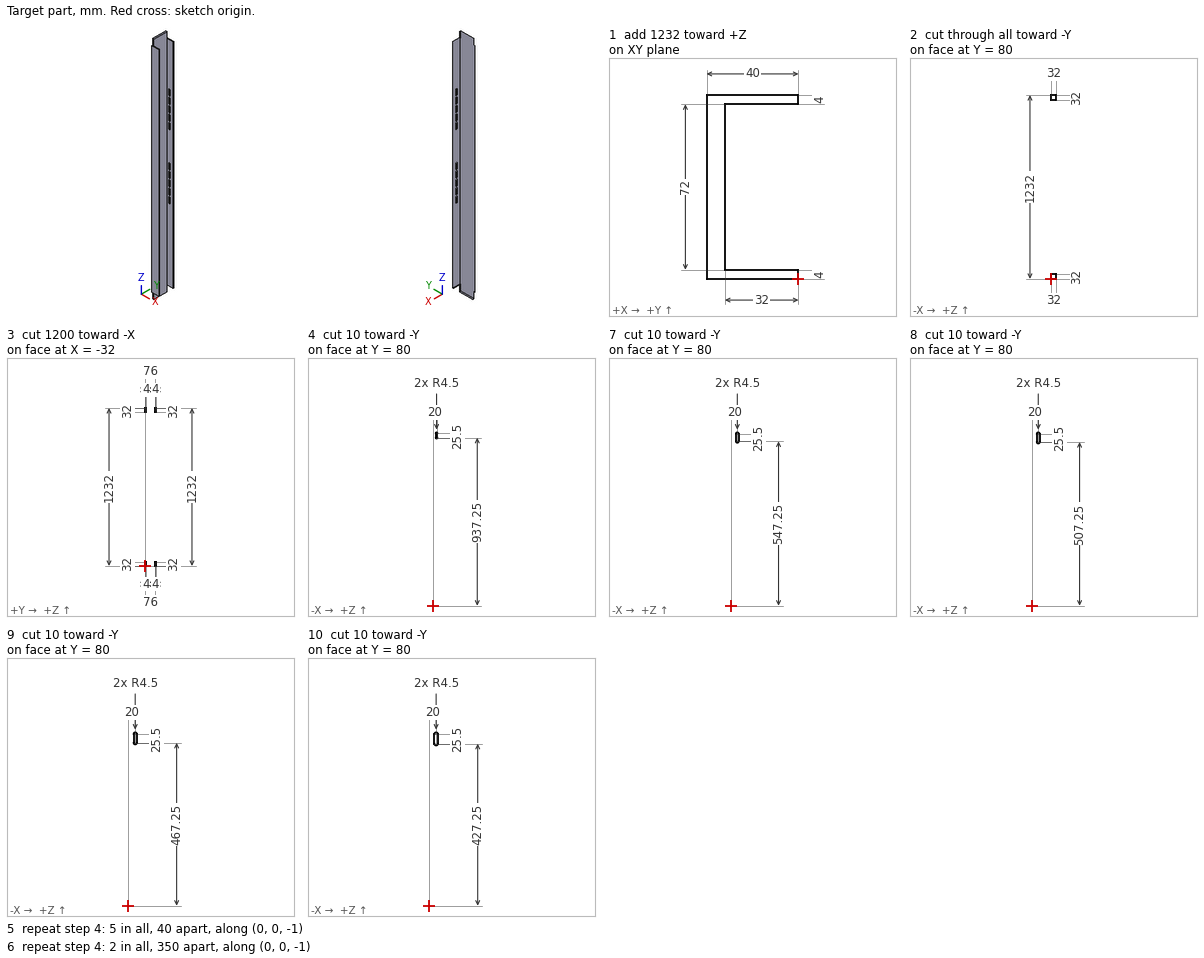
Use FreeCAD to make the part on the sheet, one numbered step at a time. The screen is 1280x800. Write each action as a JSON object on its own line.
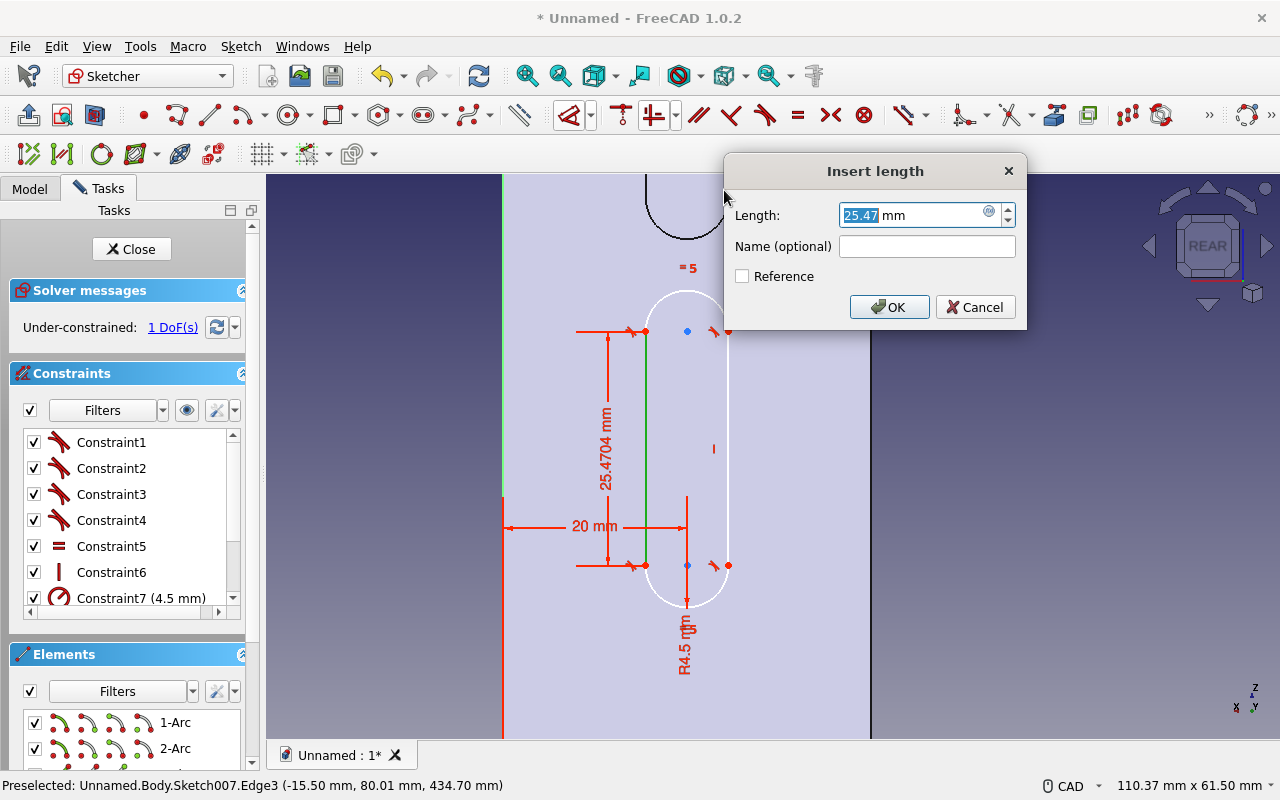
{"action": "type", "text": "25.5"}
{"action": "key", "text": "Return"}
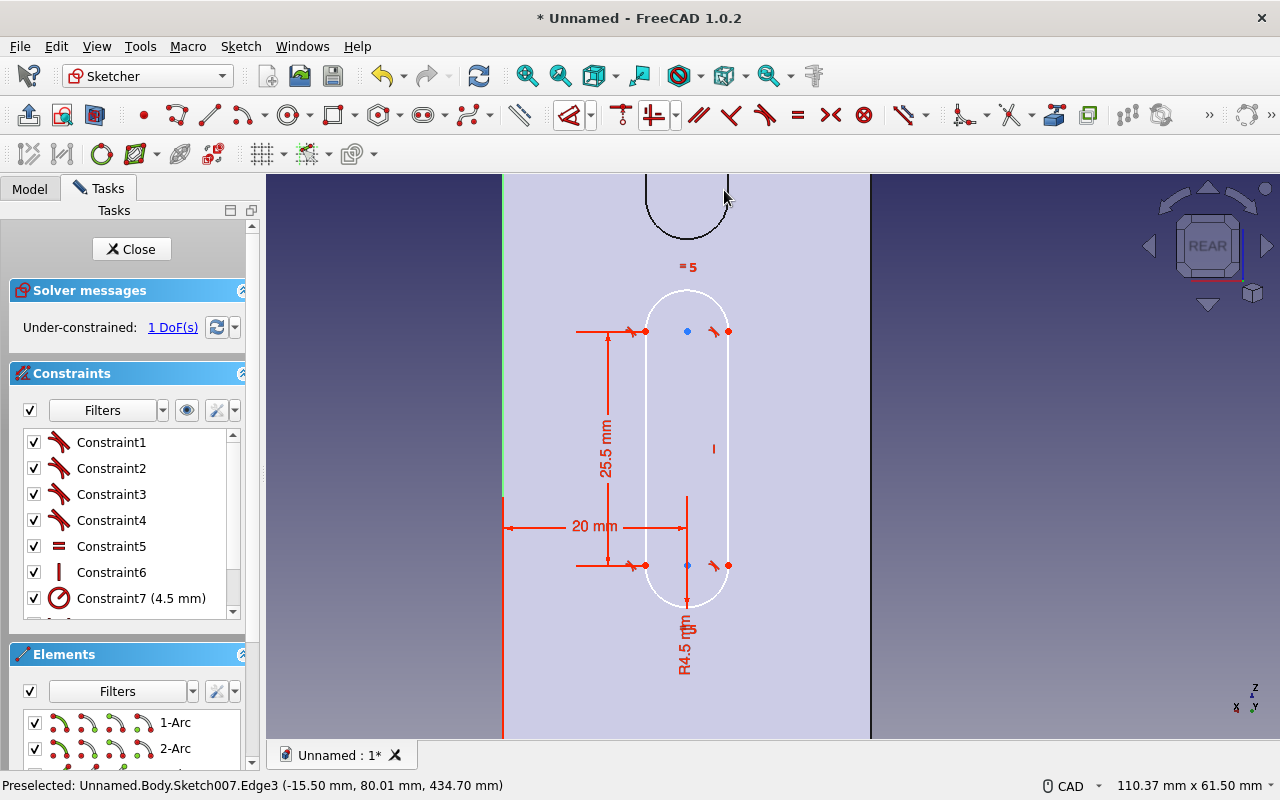
{"action": "left_click", "coordinate": [646, 566]}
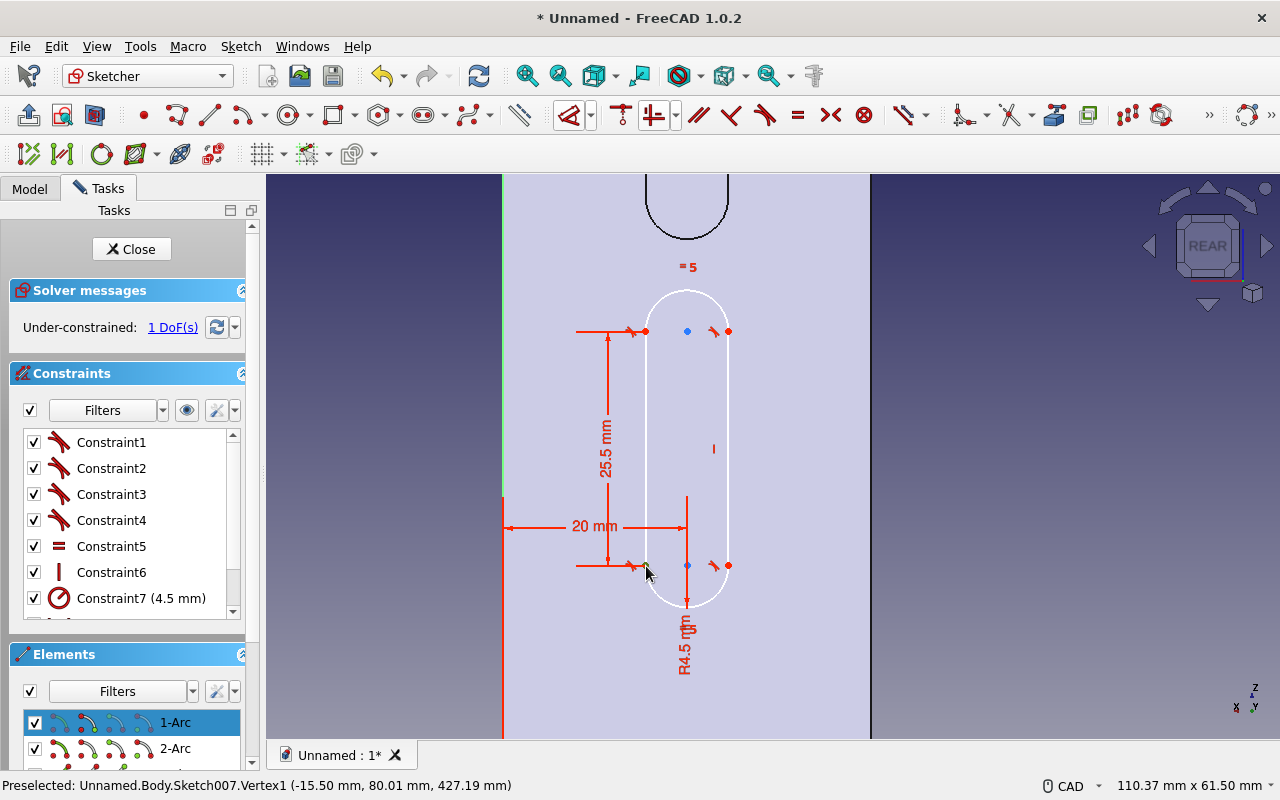
{"action": "left_click", "coordinate": [590, 116]}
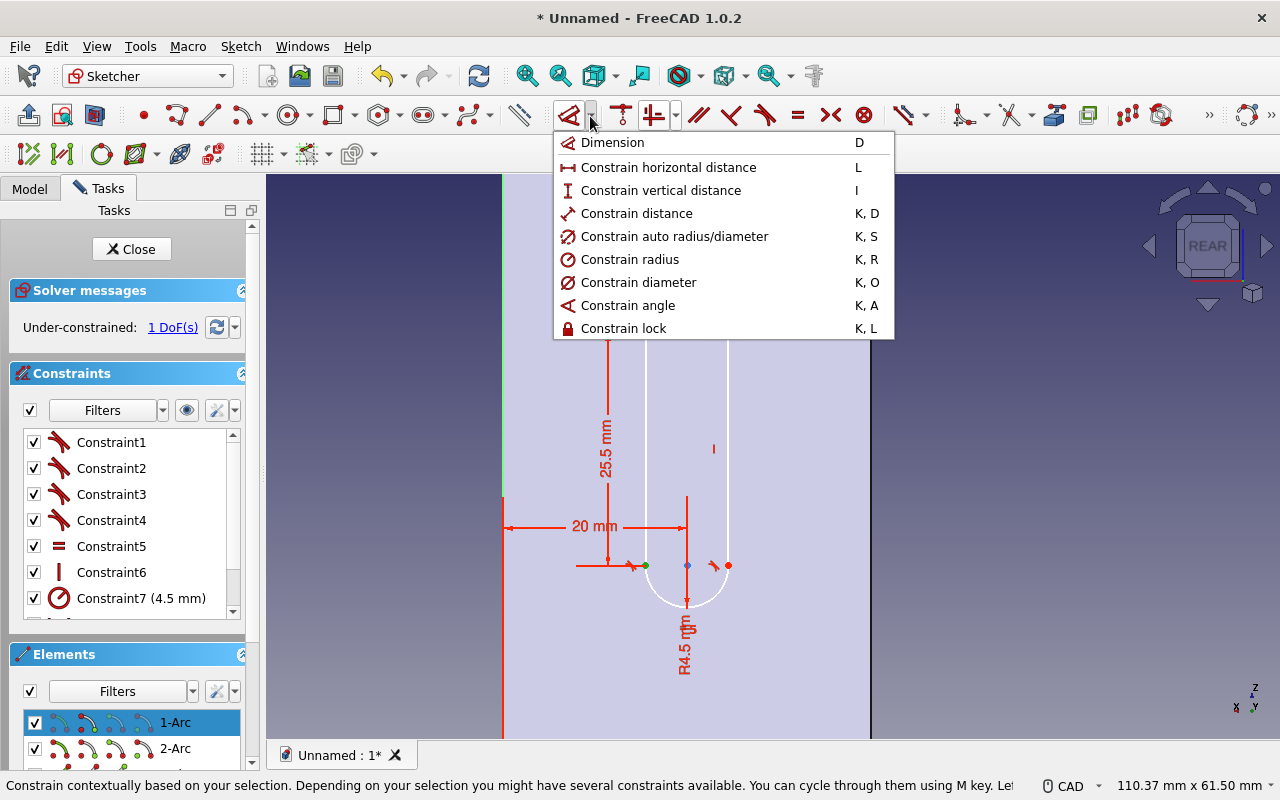
{"action": "left_click", "coordinate": [724, 190]}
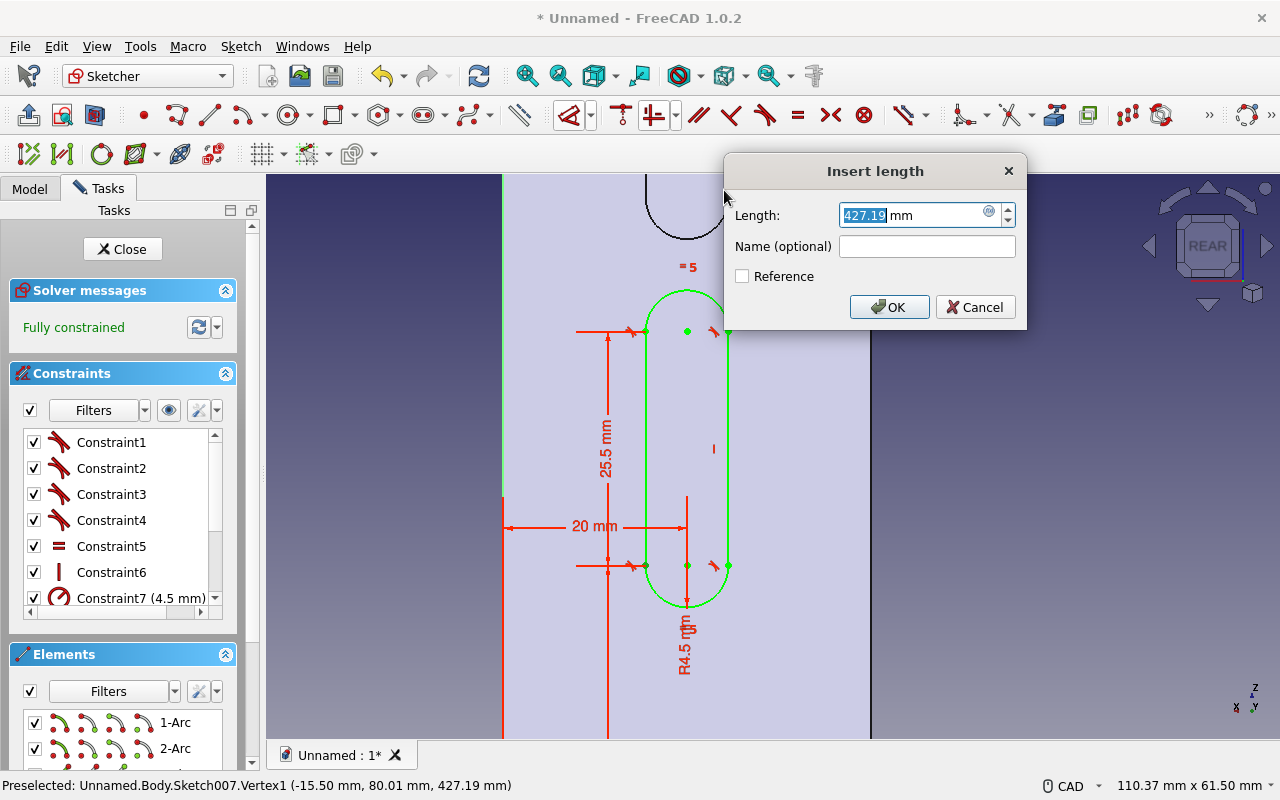
{"action": "type", "text": "427.25"}
{"action": "key", "text": "Return"}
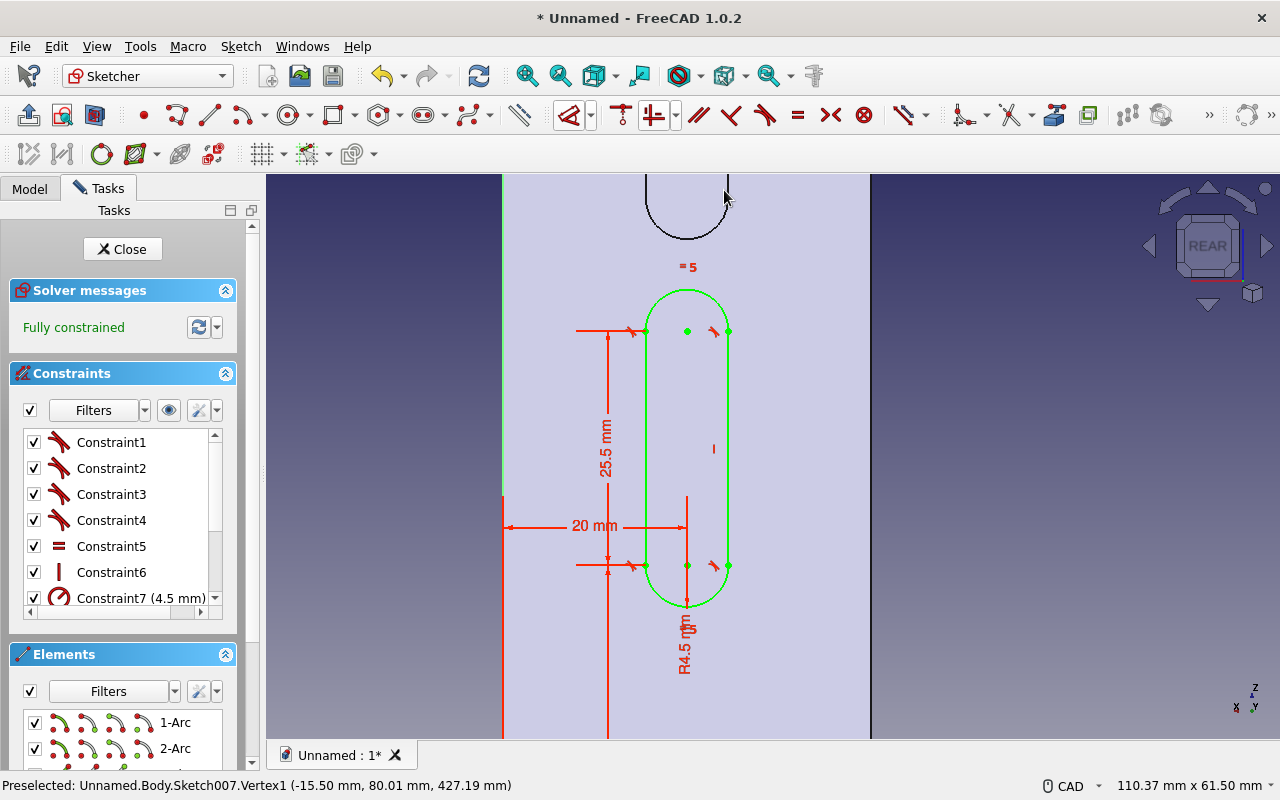
{"action": "left_click", "coordinate": [123, 249]}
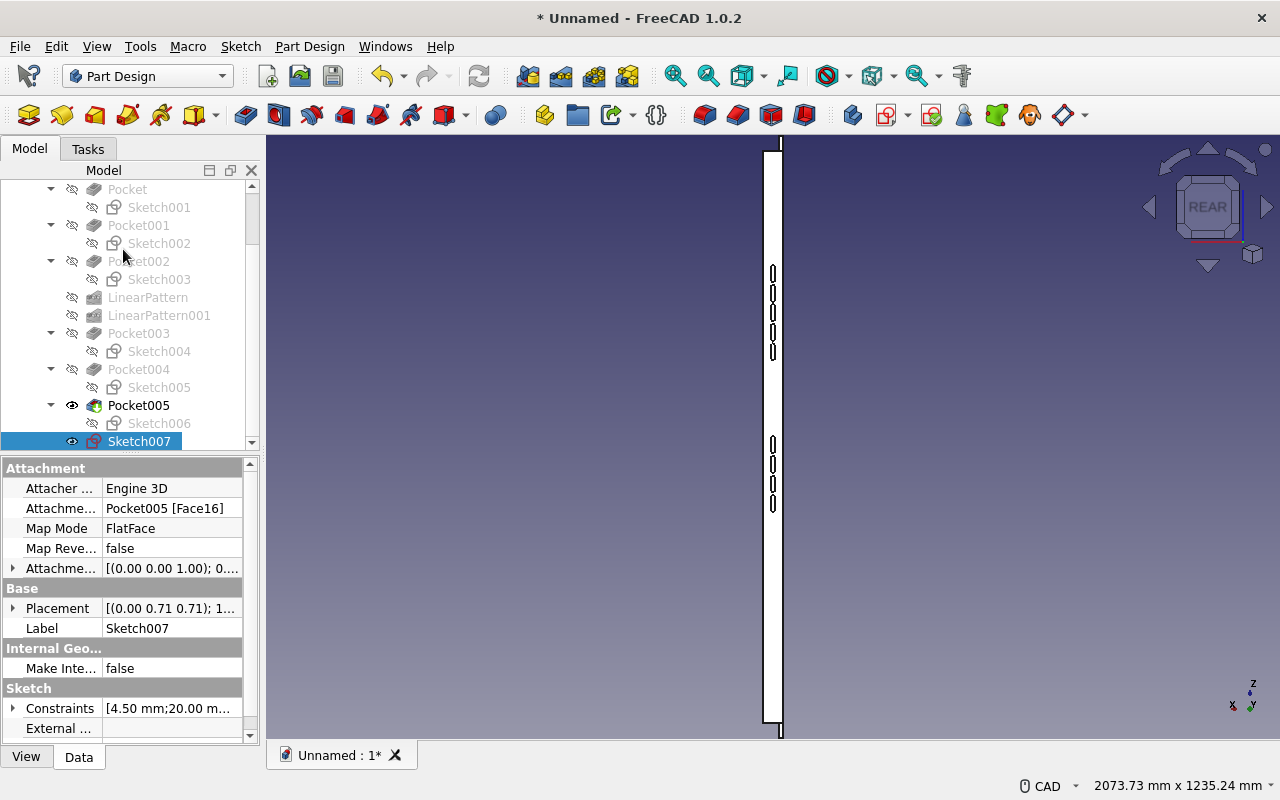
{"action": "left_click", "coordinate": [246, 116]}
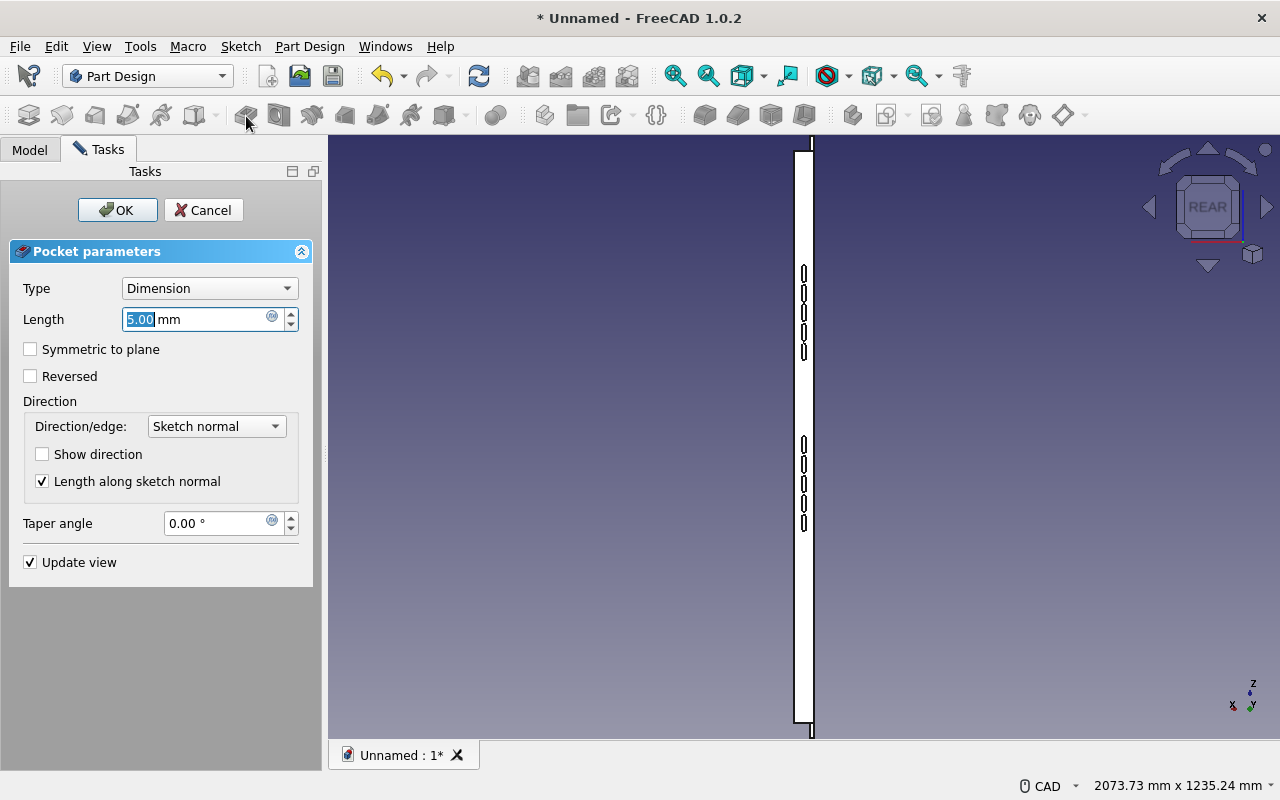
{"action": "type", "text": "10"}
{"action": "key", "text": "Tab"}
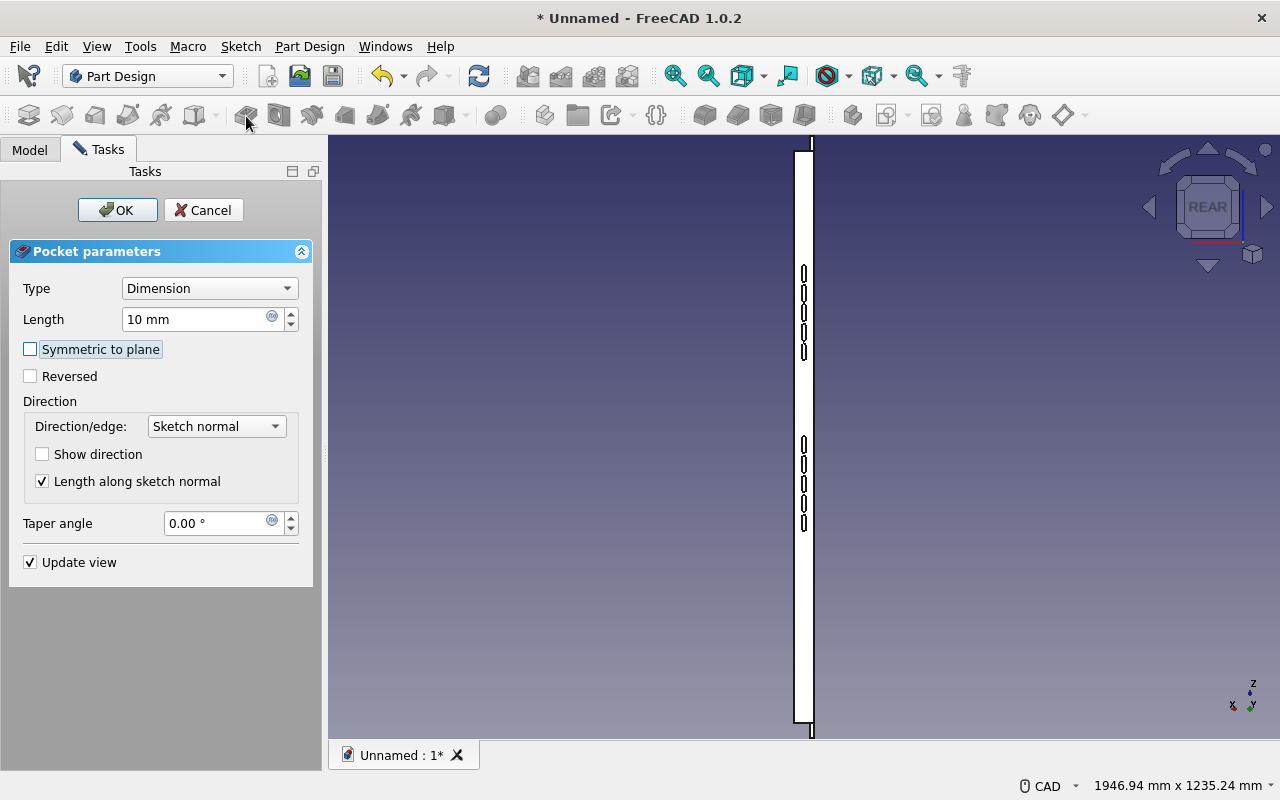
{"action": "left_click", "coordinate": [118, 210]}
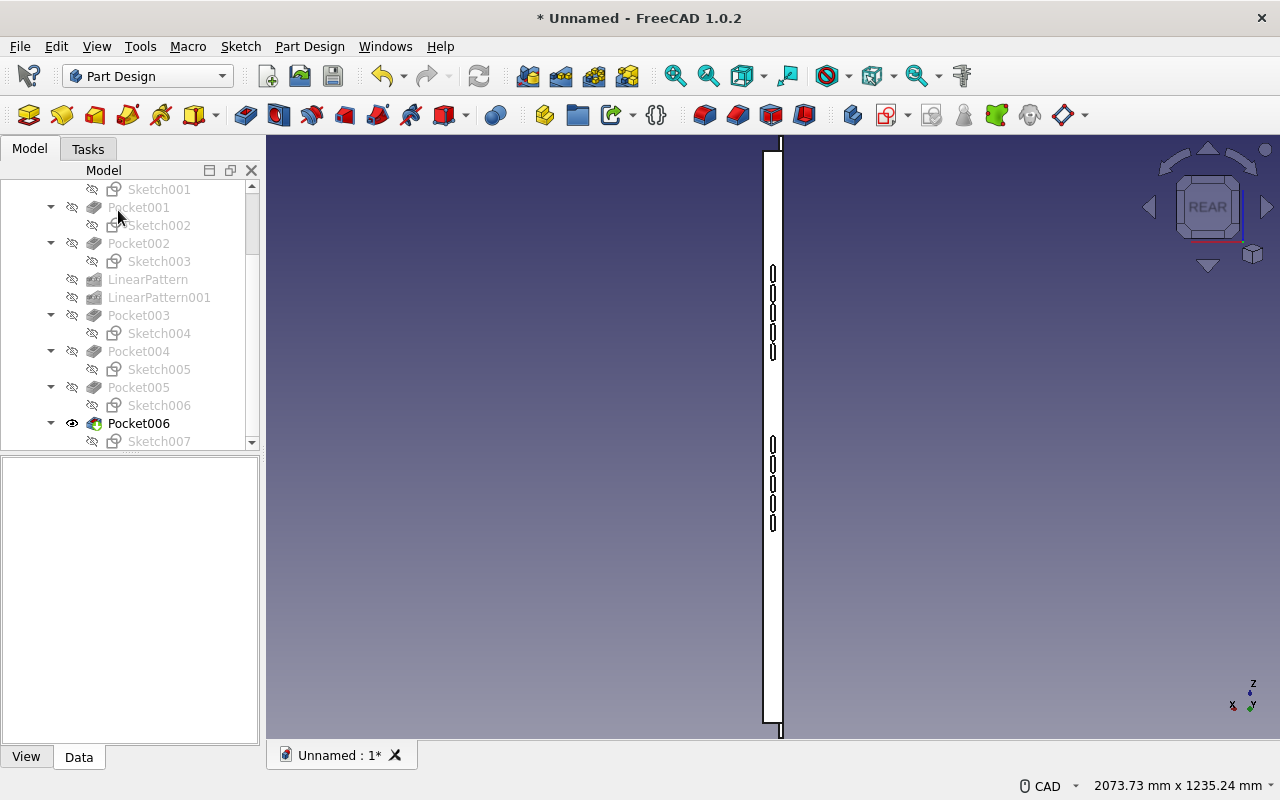
{"action": "key", "text": "0"}